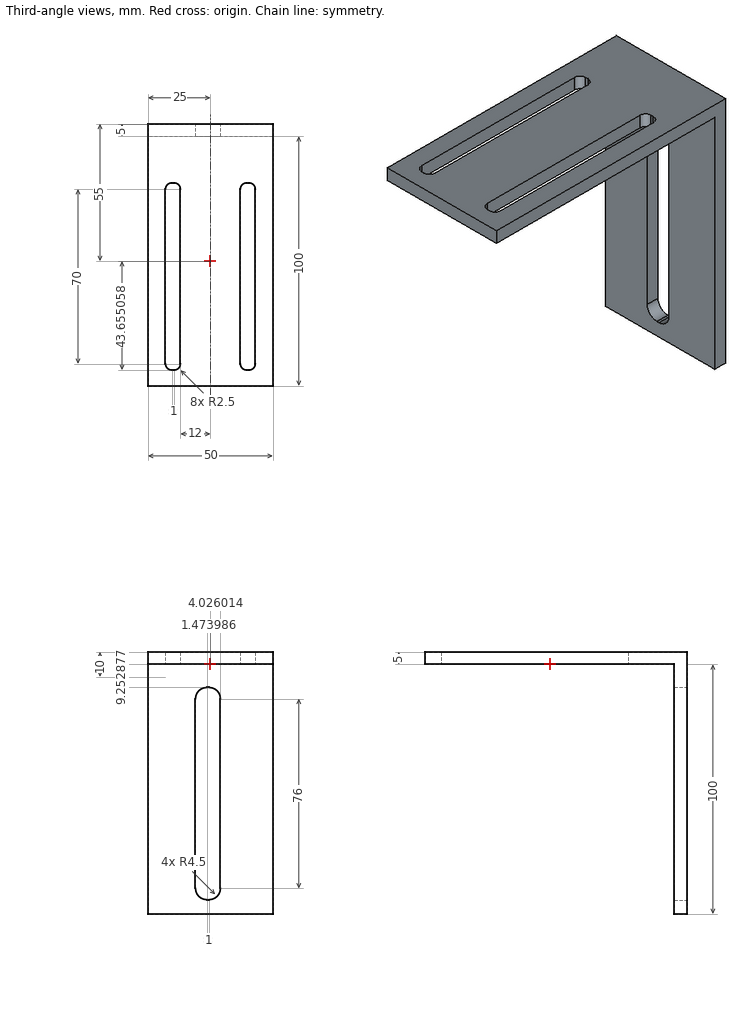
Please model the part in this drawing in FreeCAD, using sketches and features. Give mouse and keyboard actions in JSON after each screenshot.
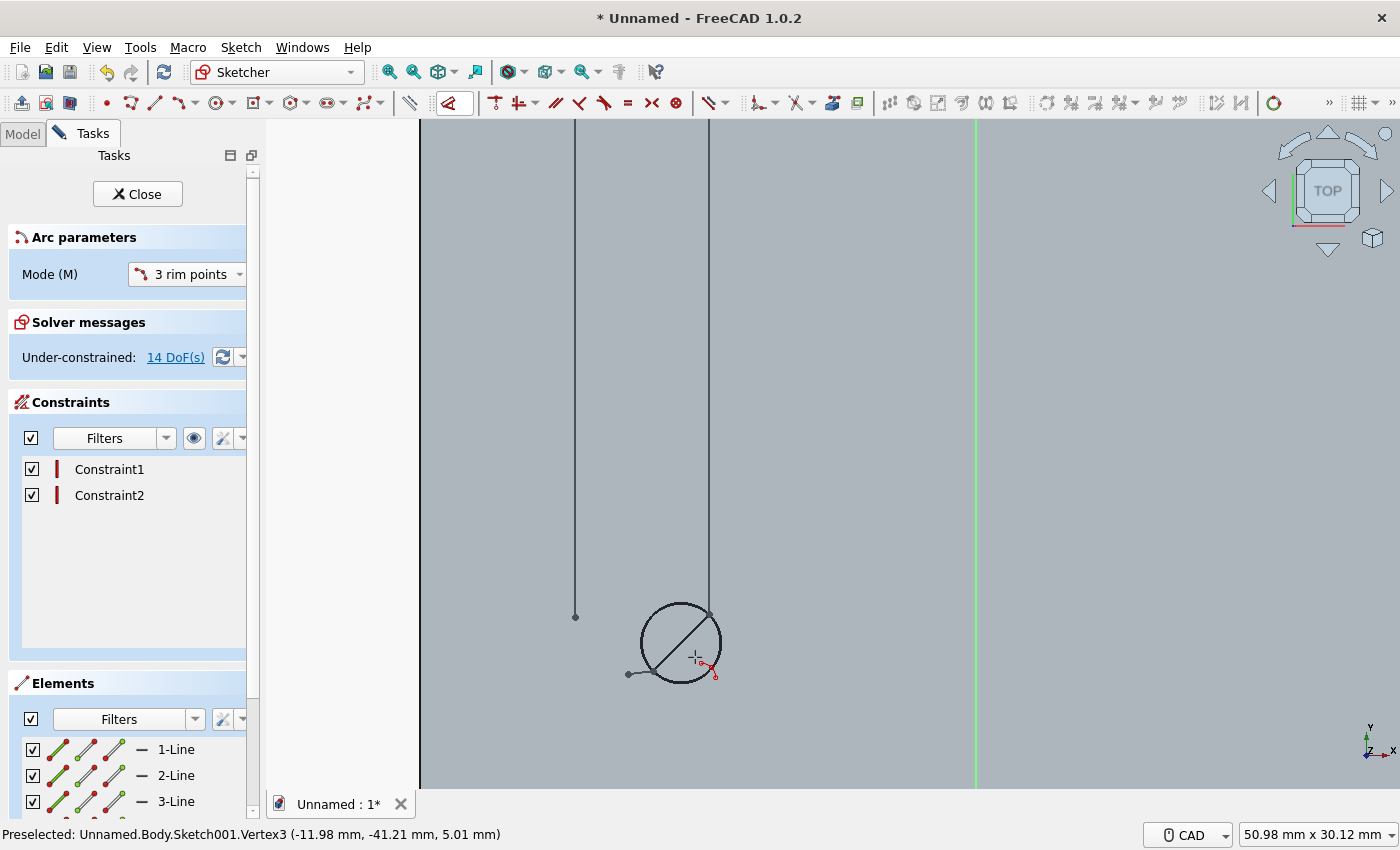
{"action": "left_click", "coordinate": [692, 653]}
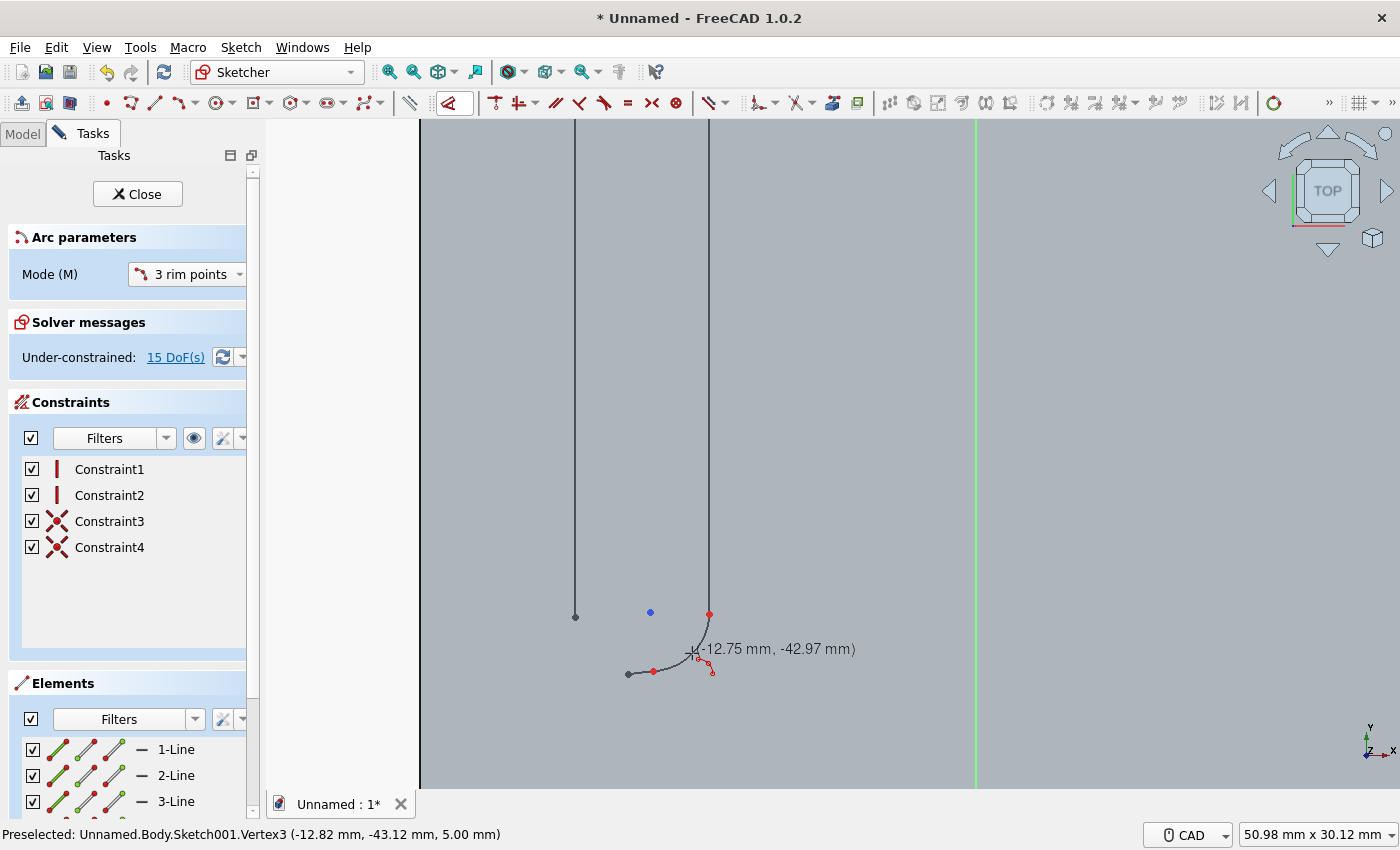
{"action": "scroll", "coordinate": [695, 657], "scroll_direction": "down", "scroll_amount": 7}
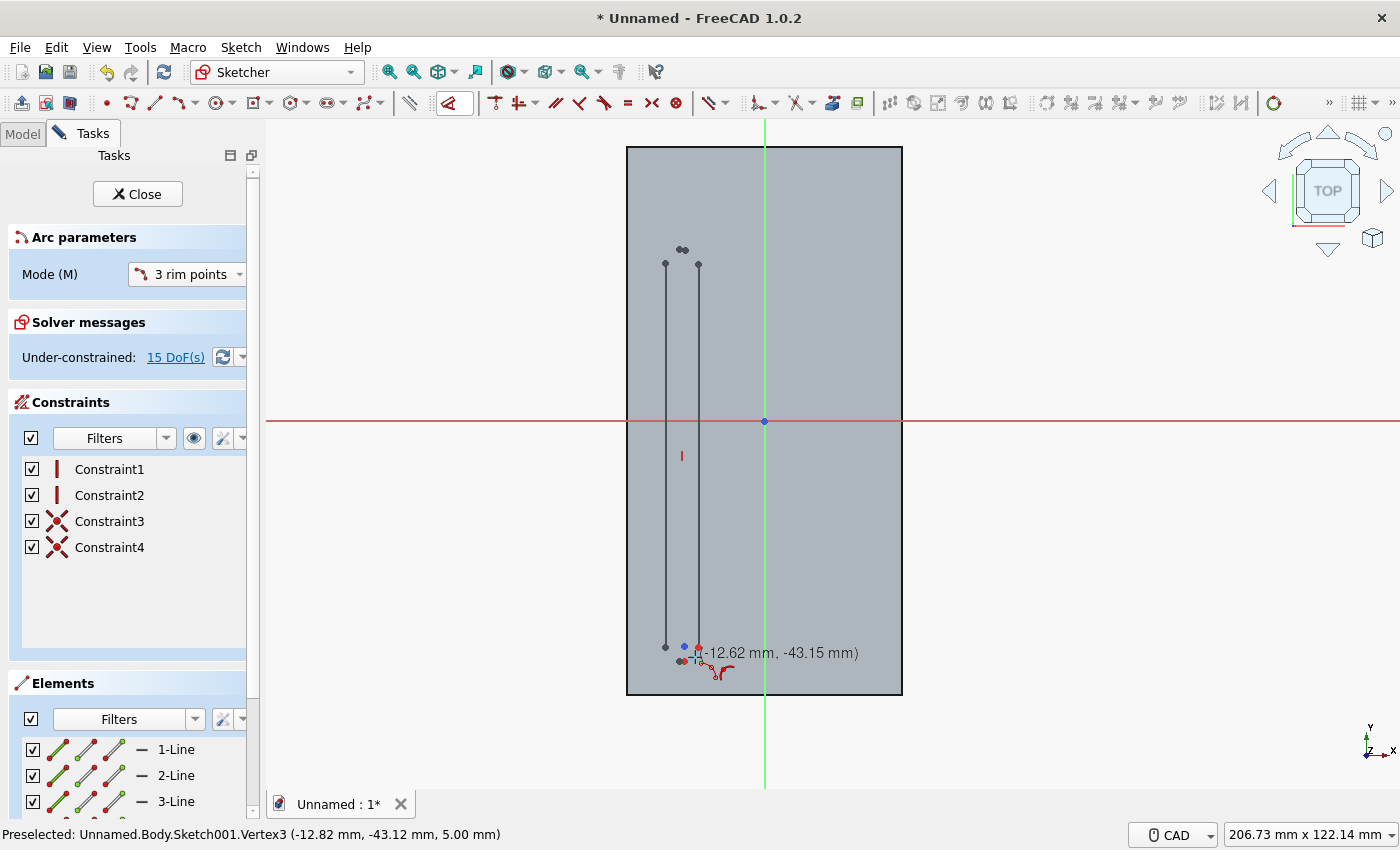
{"action": "left_click", "coordinate": [699, 264]}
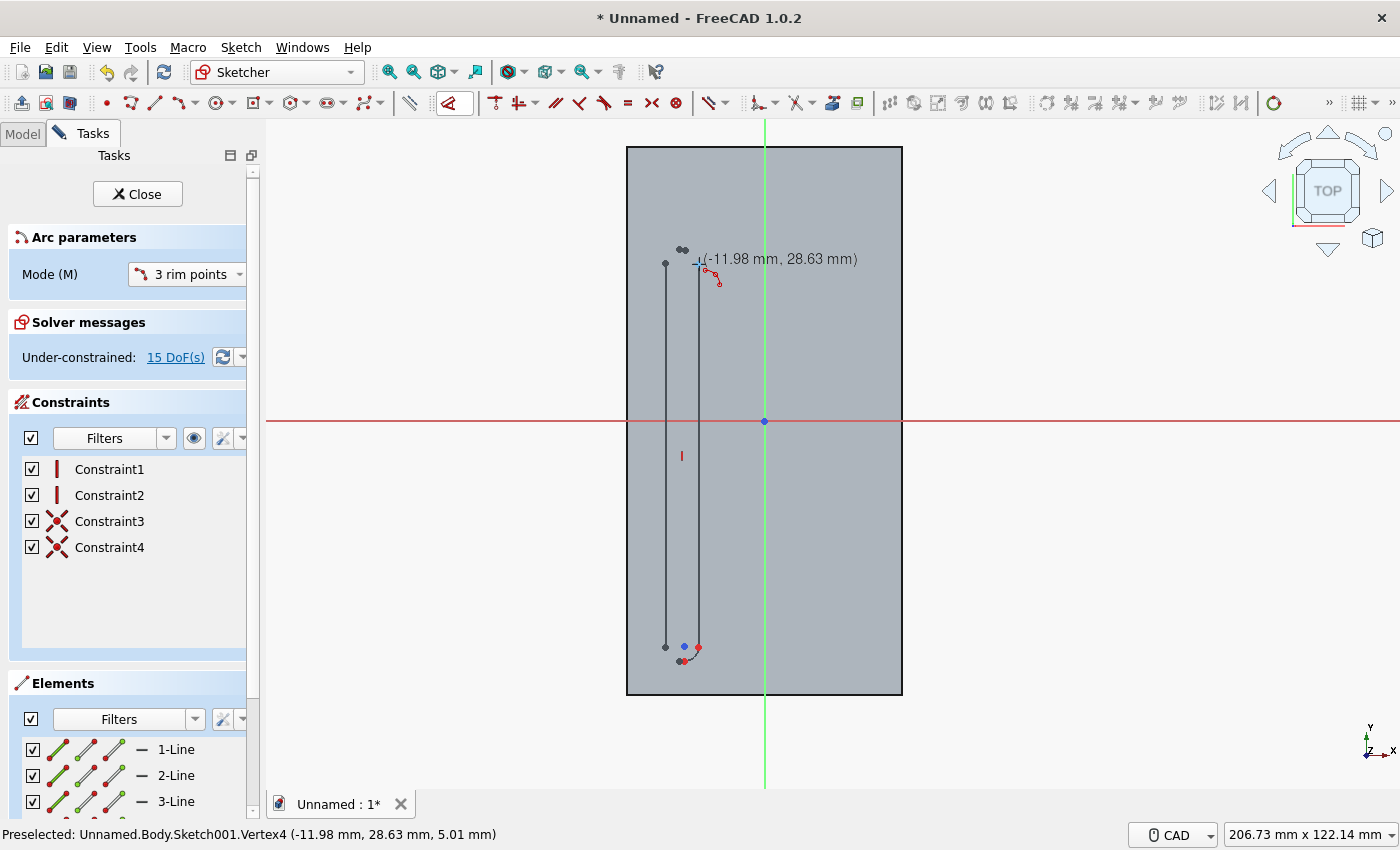
{"action": "scroll", "coordinate": [685, 249], "scroll_direction": "up", "scroll_amount": 9}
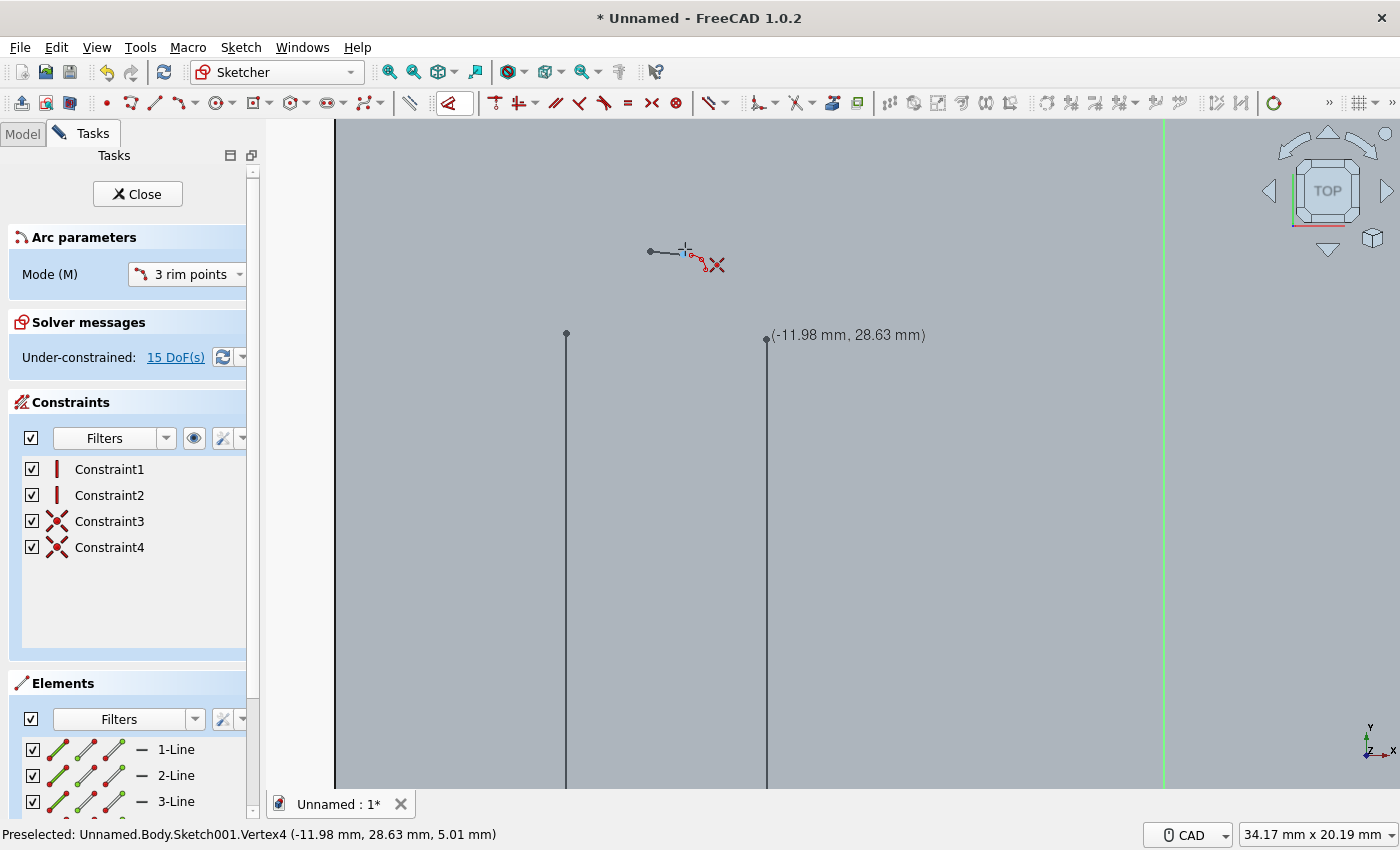
{"action": "left_click", "coordinate": [683, 255]}
{"action": "left_click", "coordinate": [742, 274]}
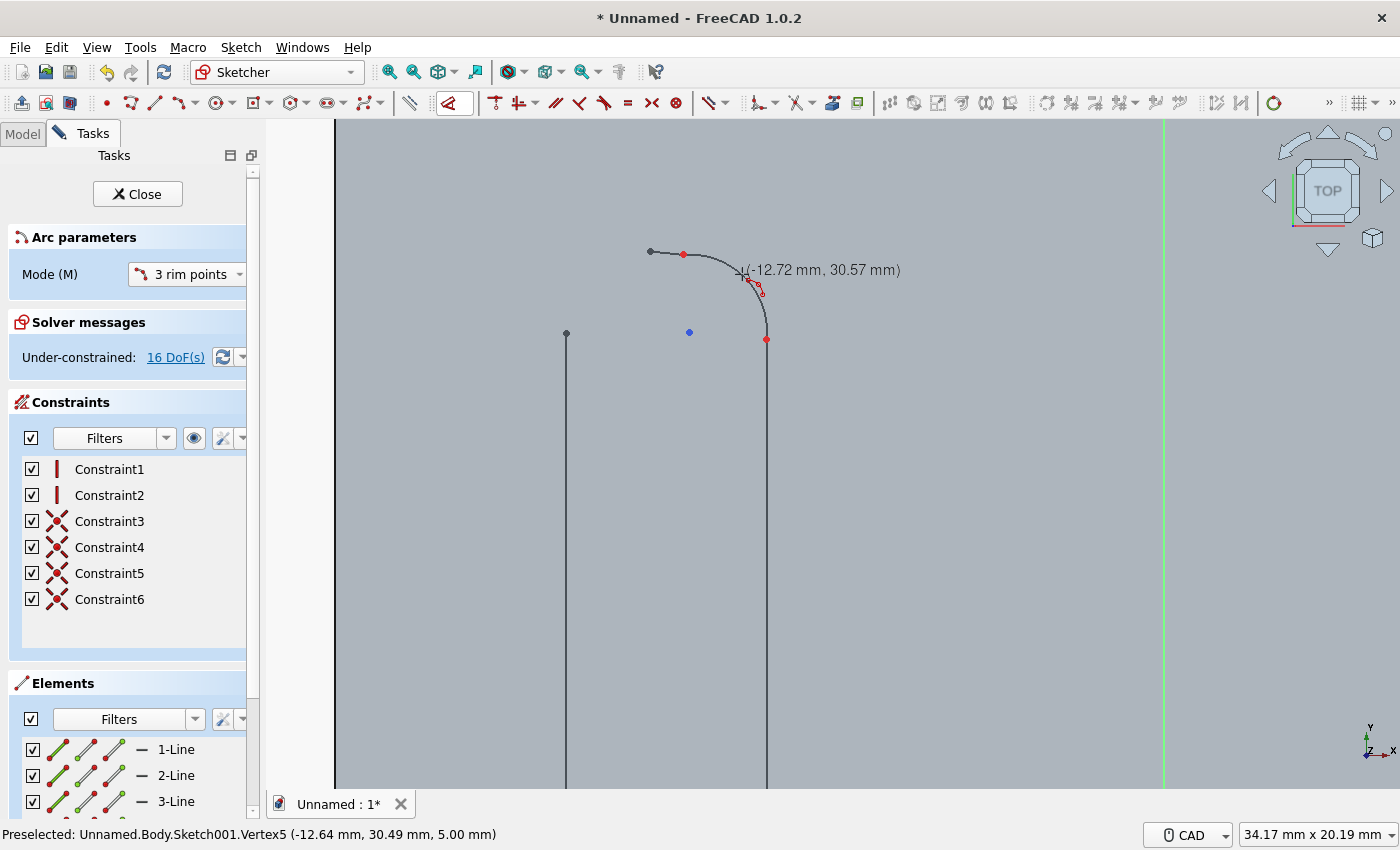
{"action": "left_click", "coordinate": [650, 251]}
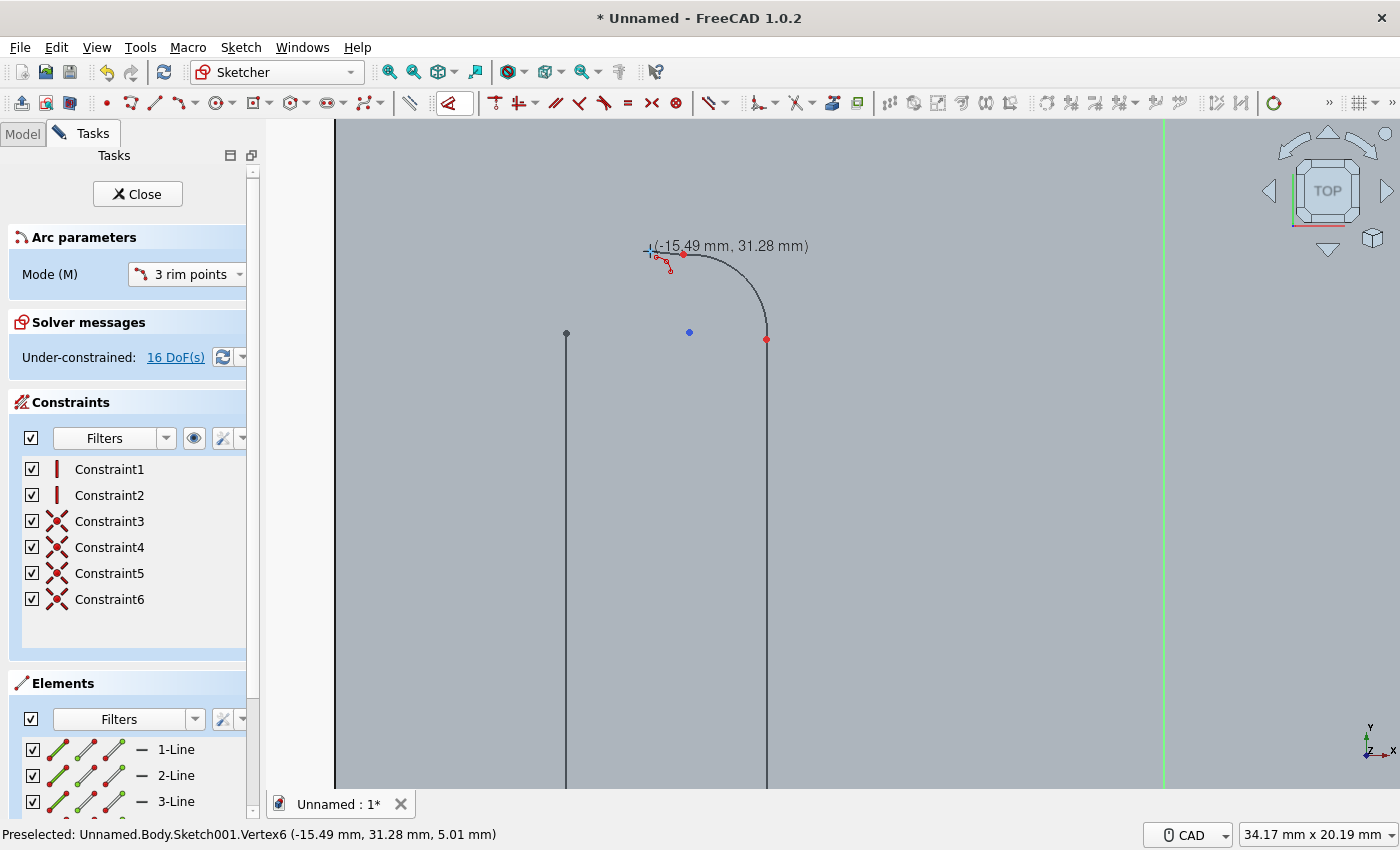
{"action": "scroll", "coordinate": [685, 248], "scroll_direction": "down", "scroll_amount": 9}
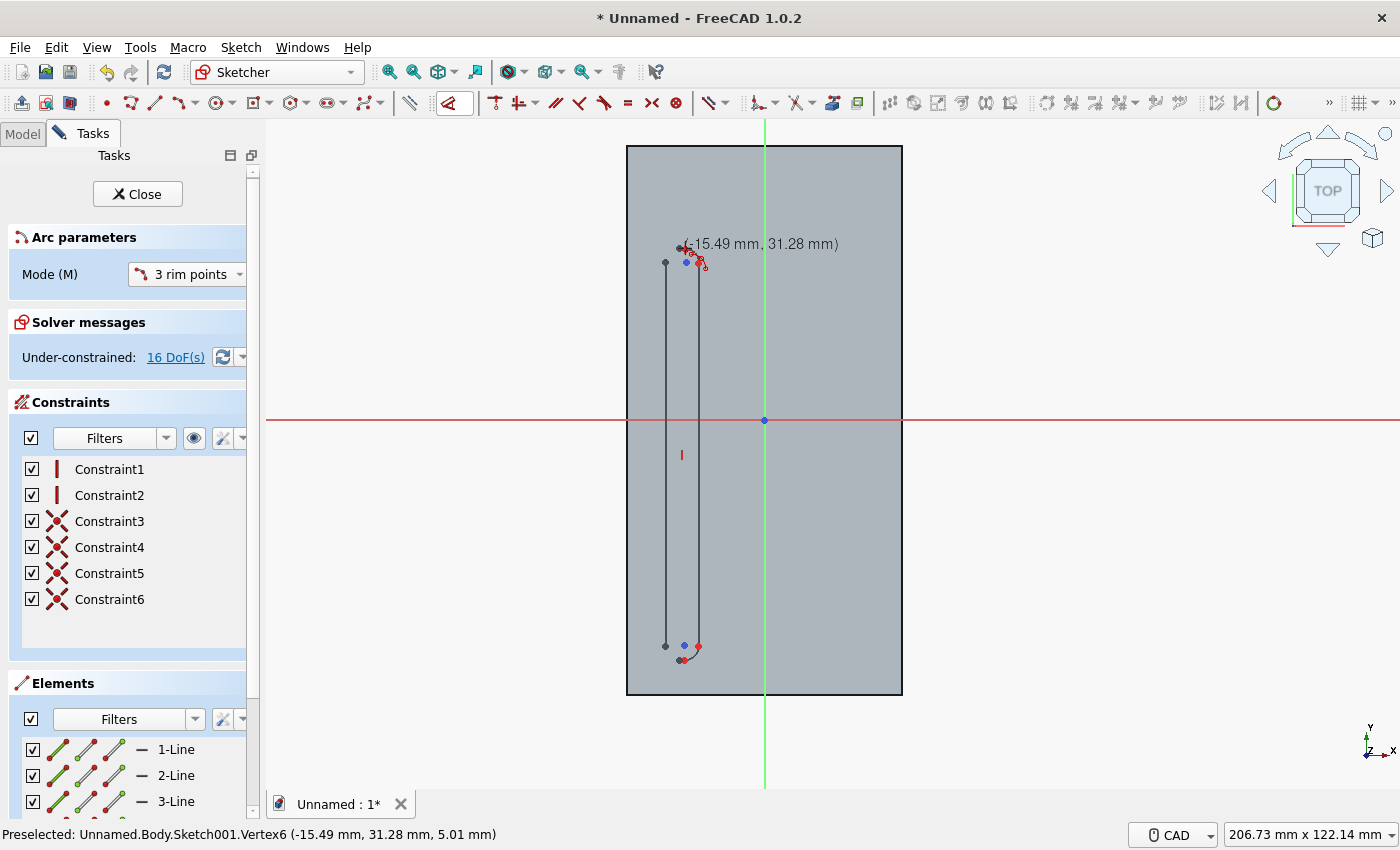
{"action": "left_click", "coordinate": [666, 262]}